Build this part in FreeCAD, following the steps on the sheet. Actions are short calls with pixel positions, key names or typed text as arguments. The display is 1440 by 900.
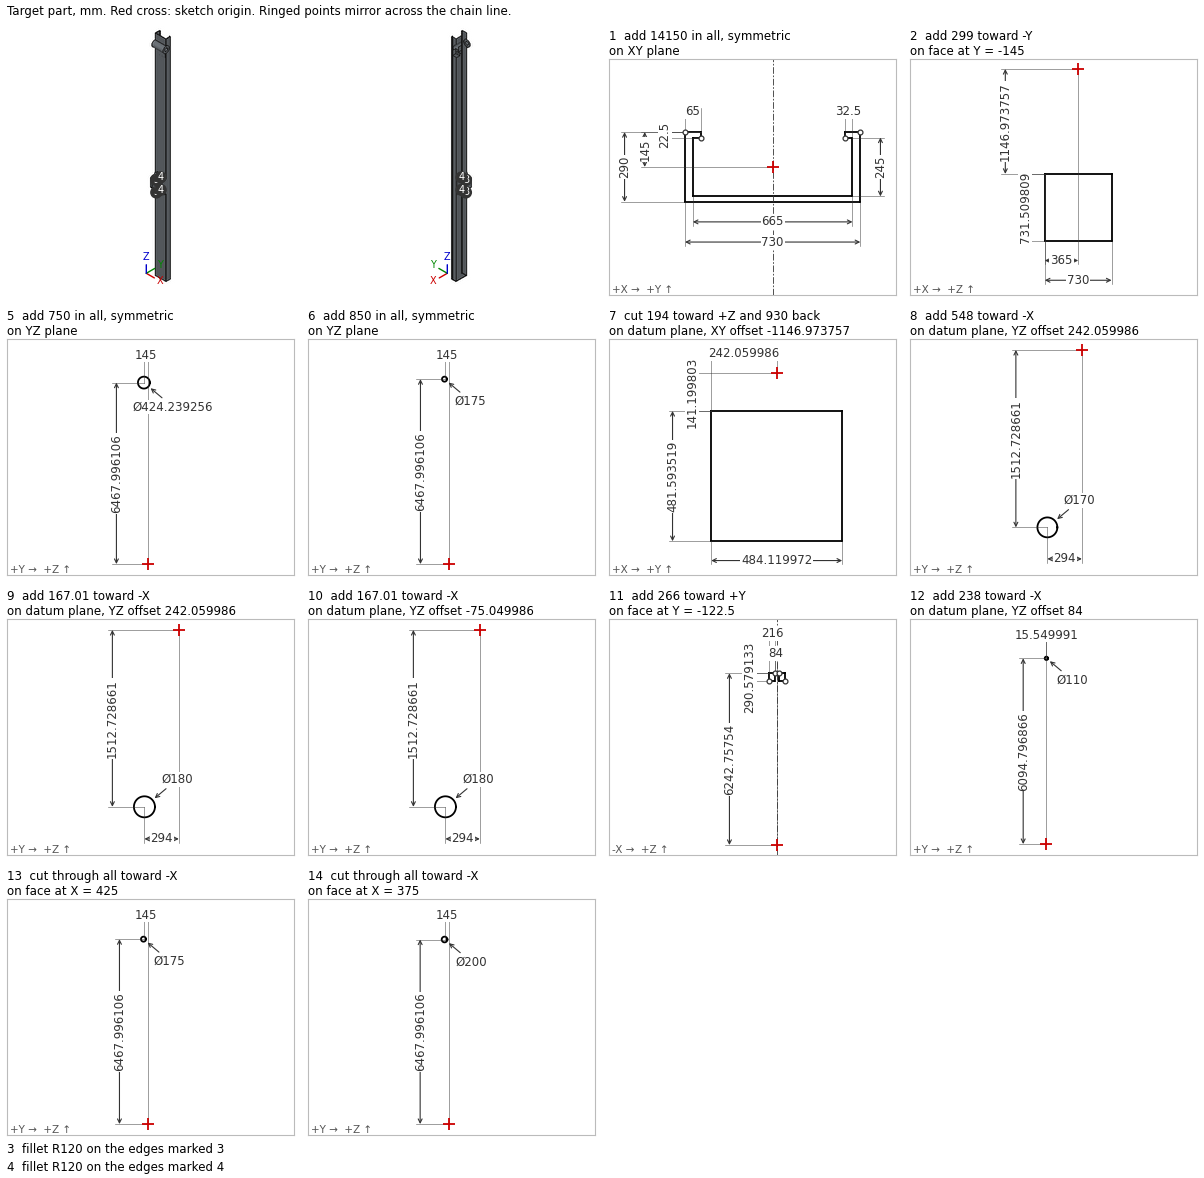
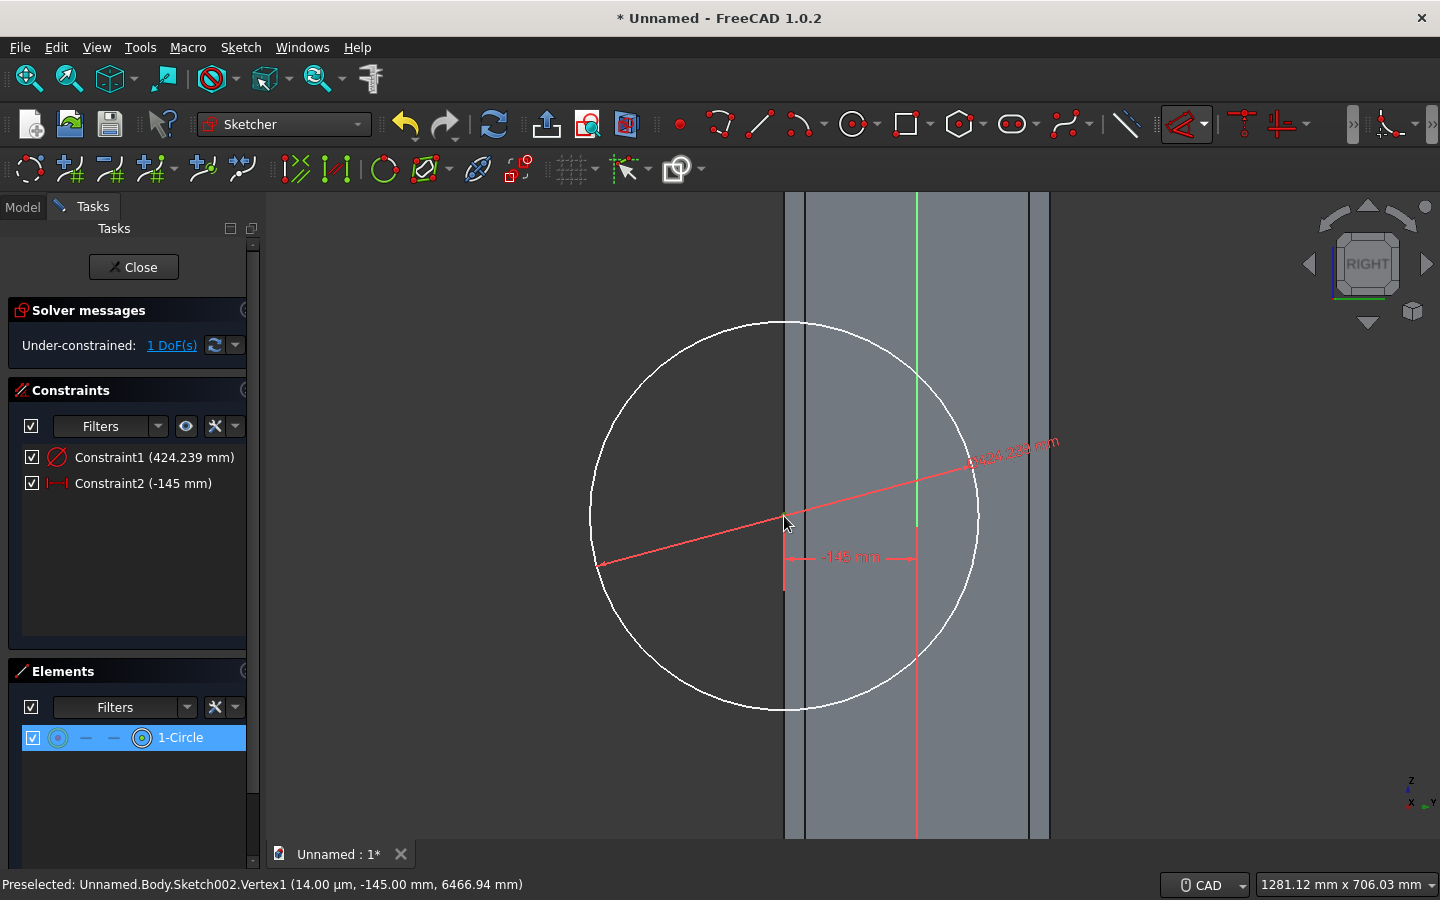
click(1206, 124)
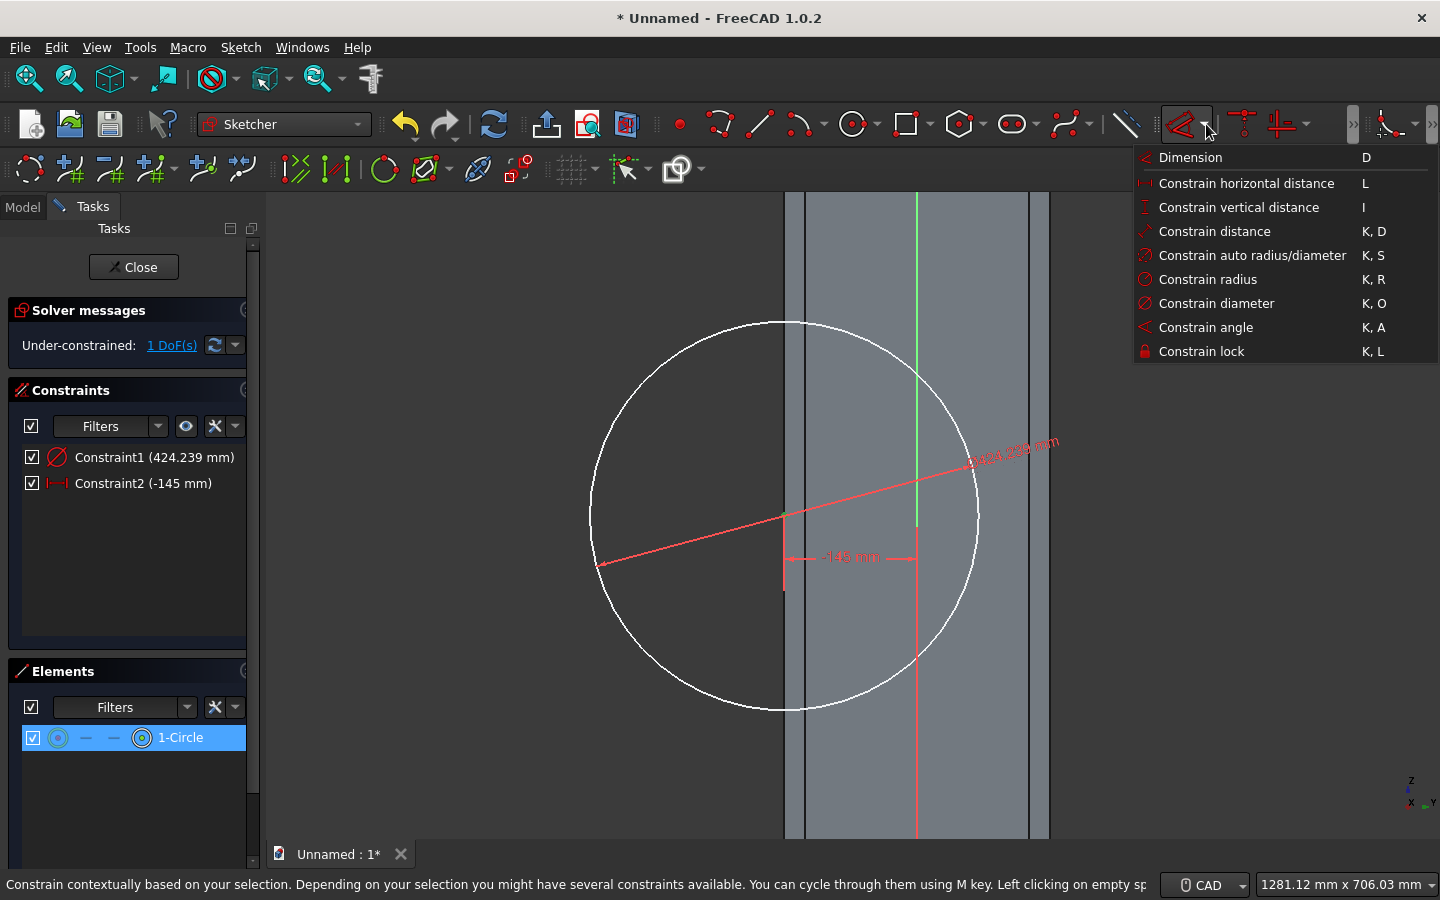
click(1286, 207)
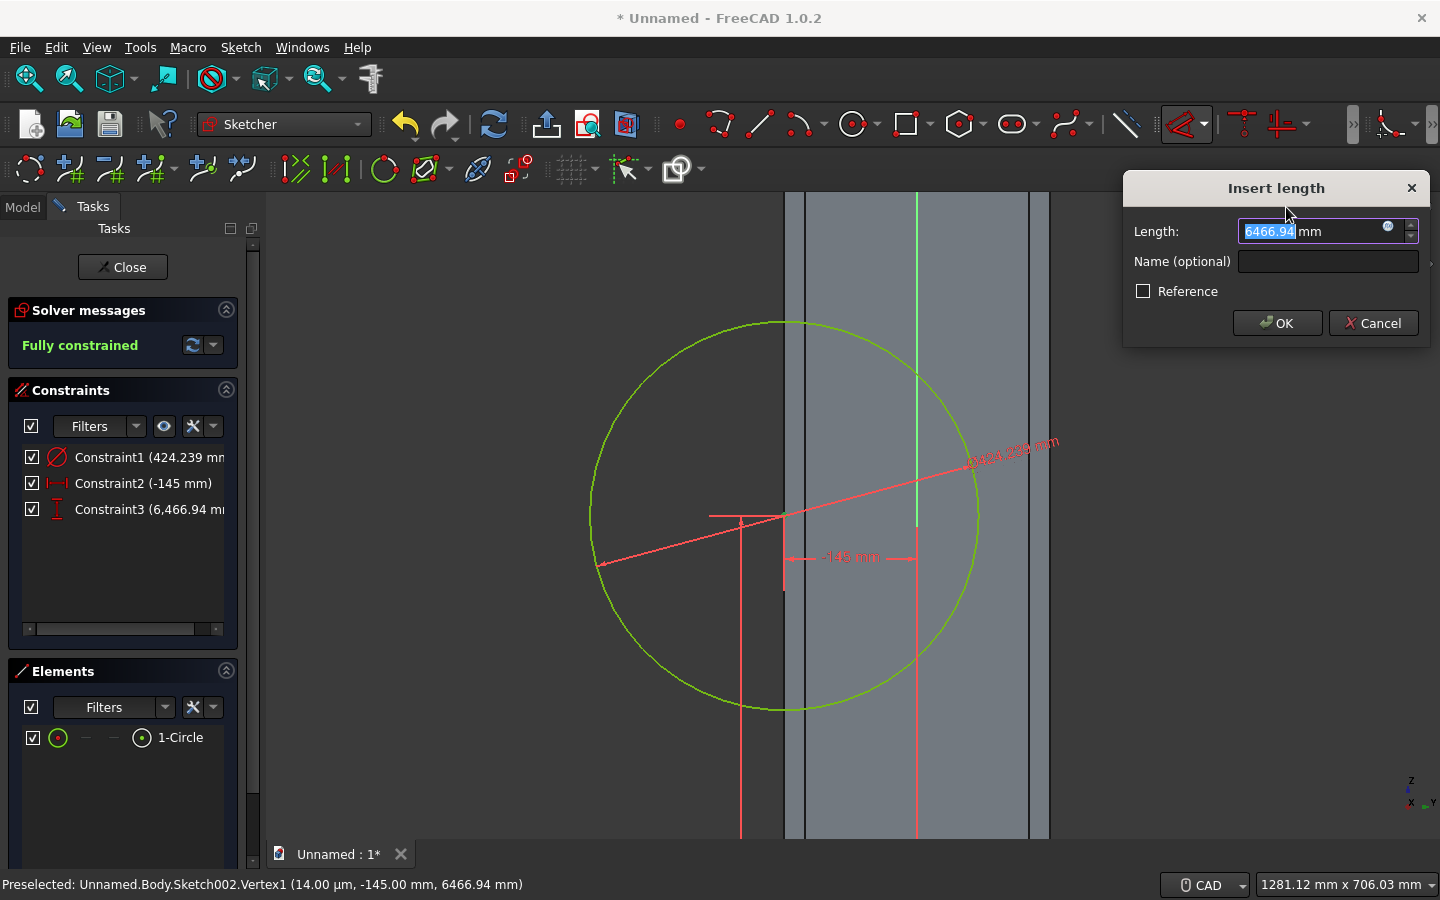
text(6467.996106)
key(Return)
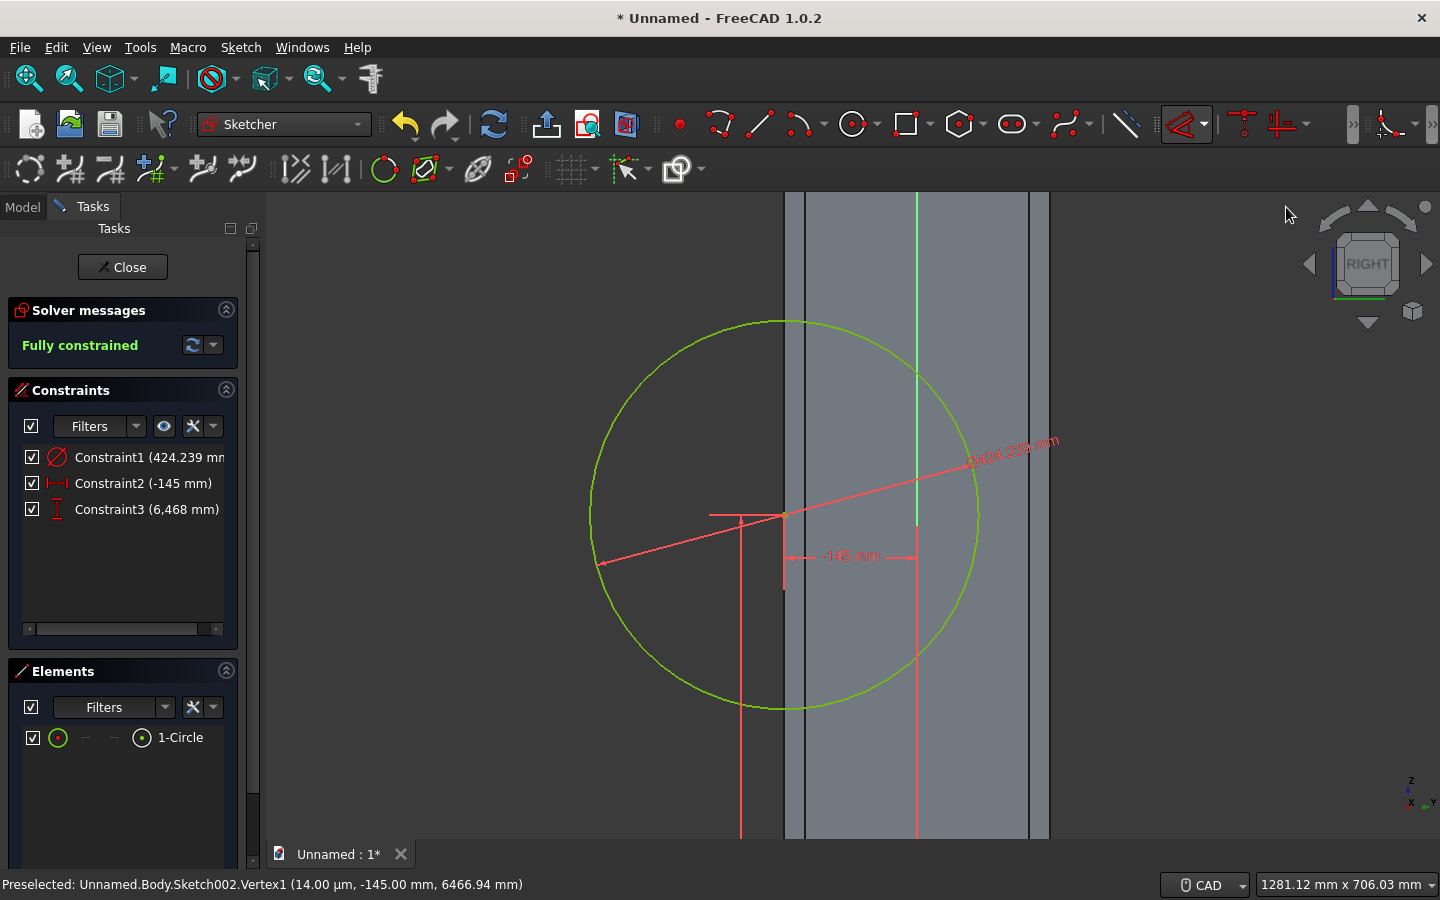
click(123, 267)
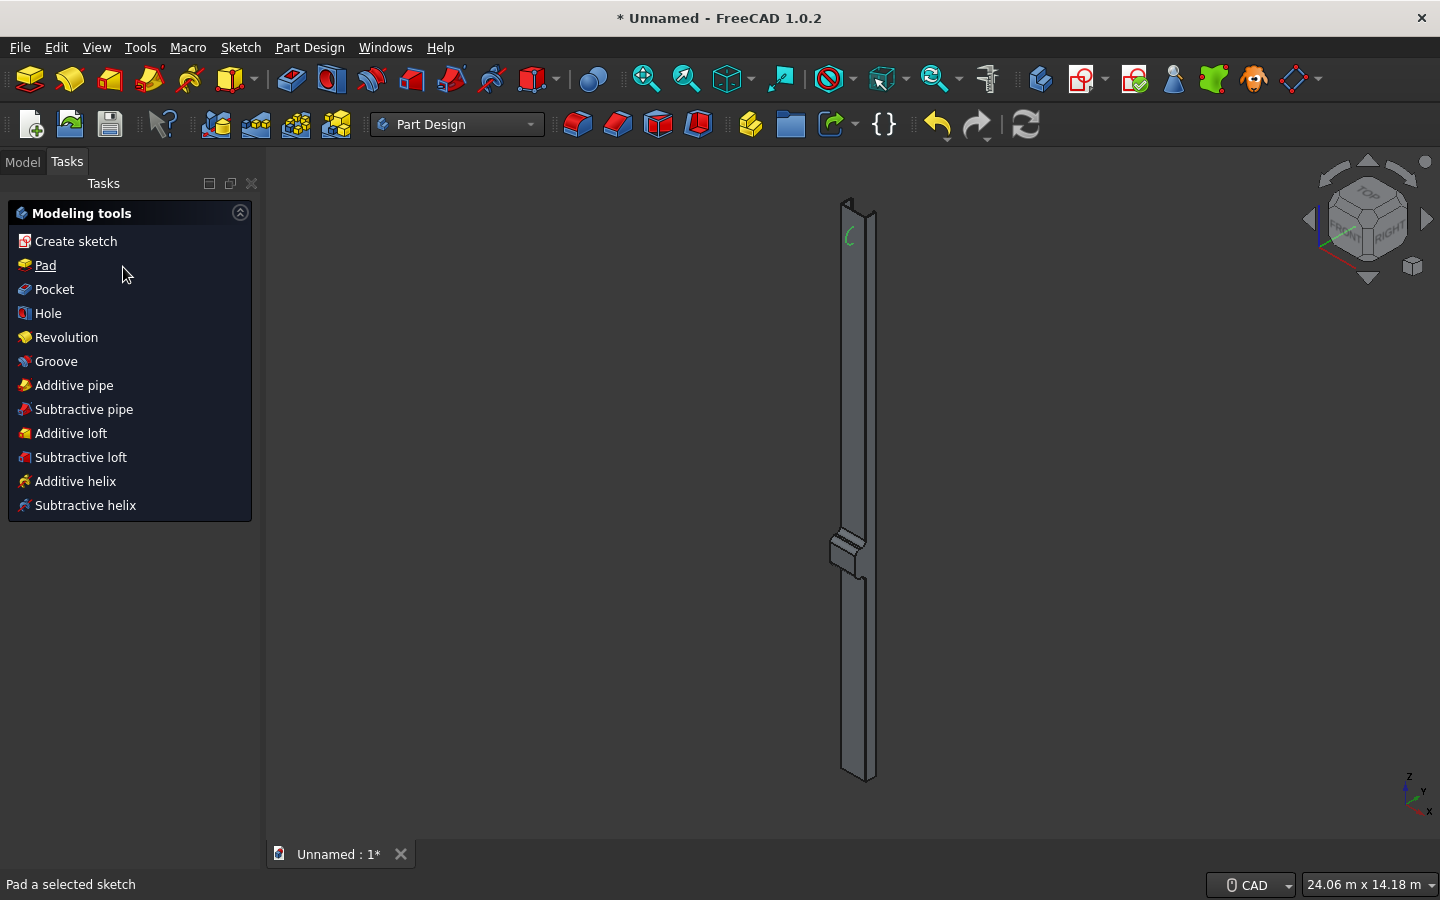
click(30, 80)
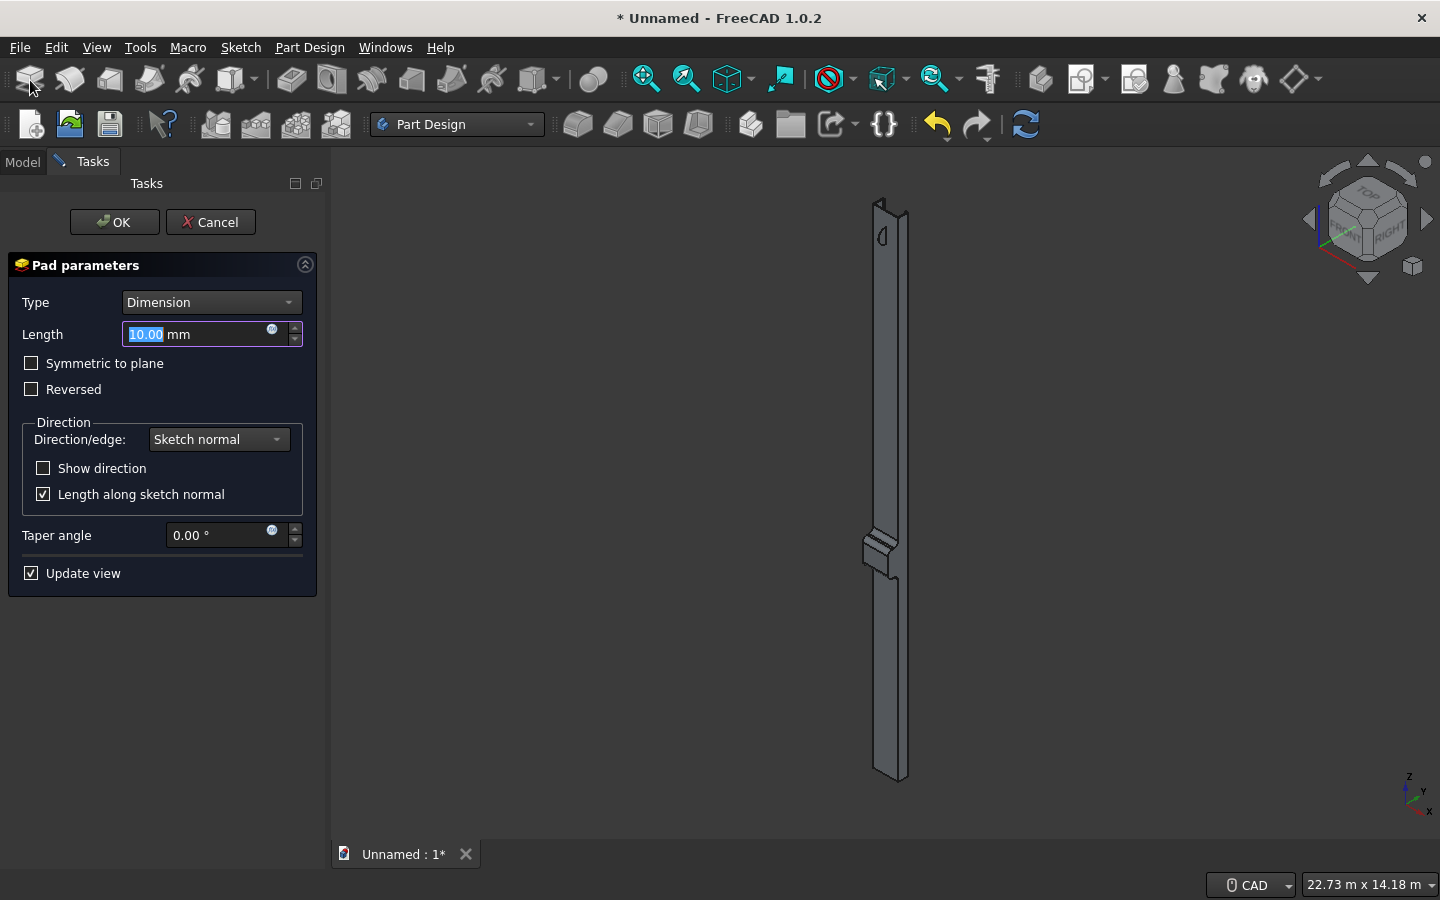
text(750)
key(Tab)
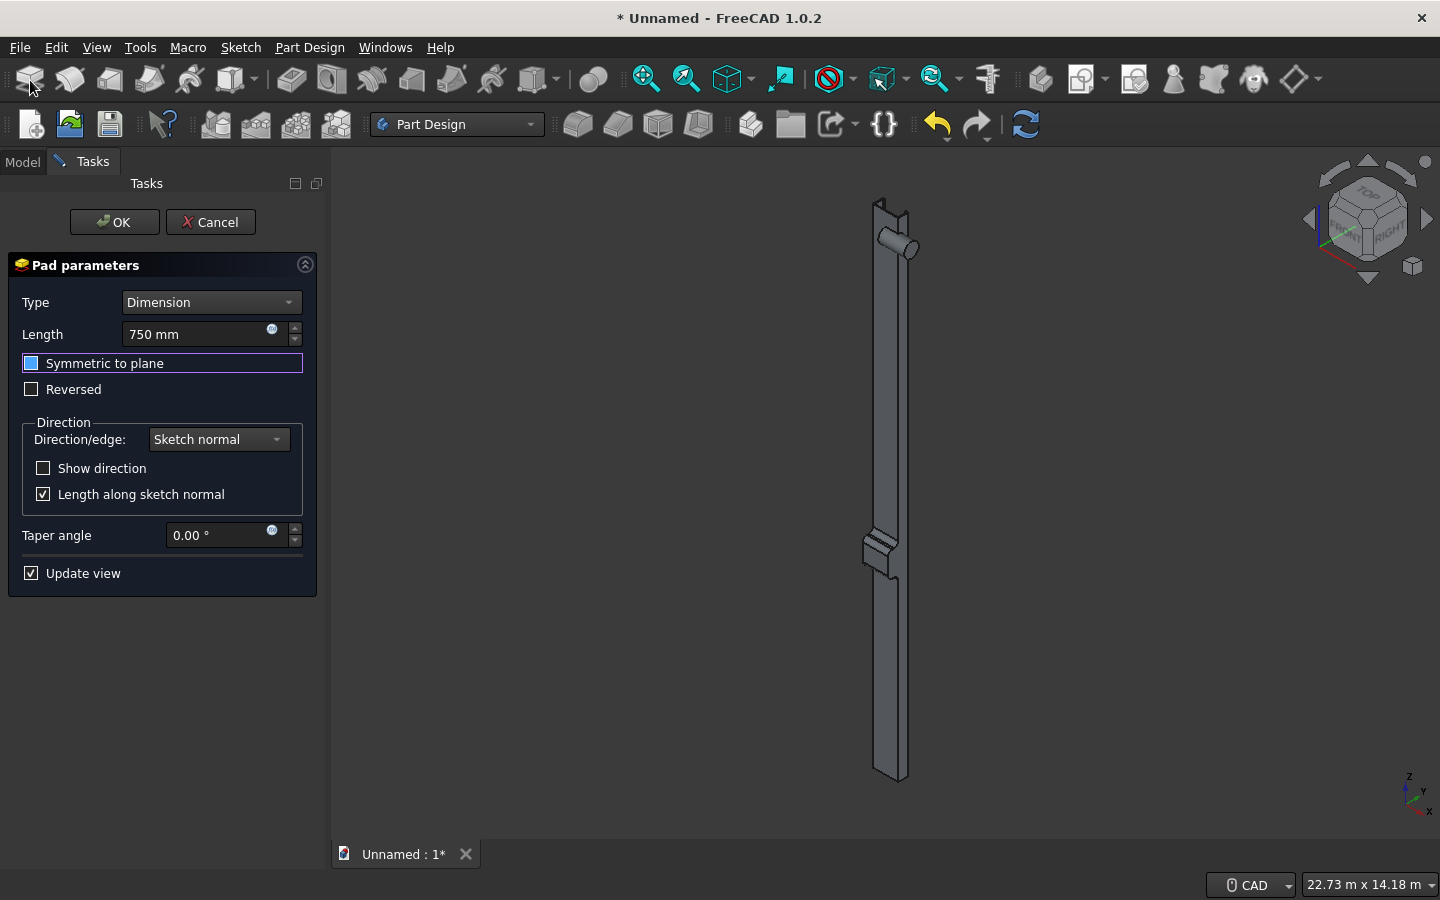
click(30, 363)